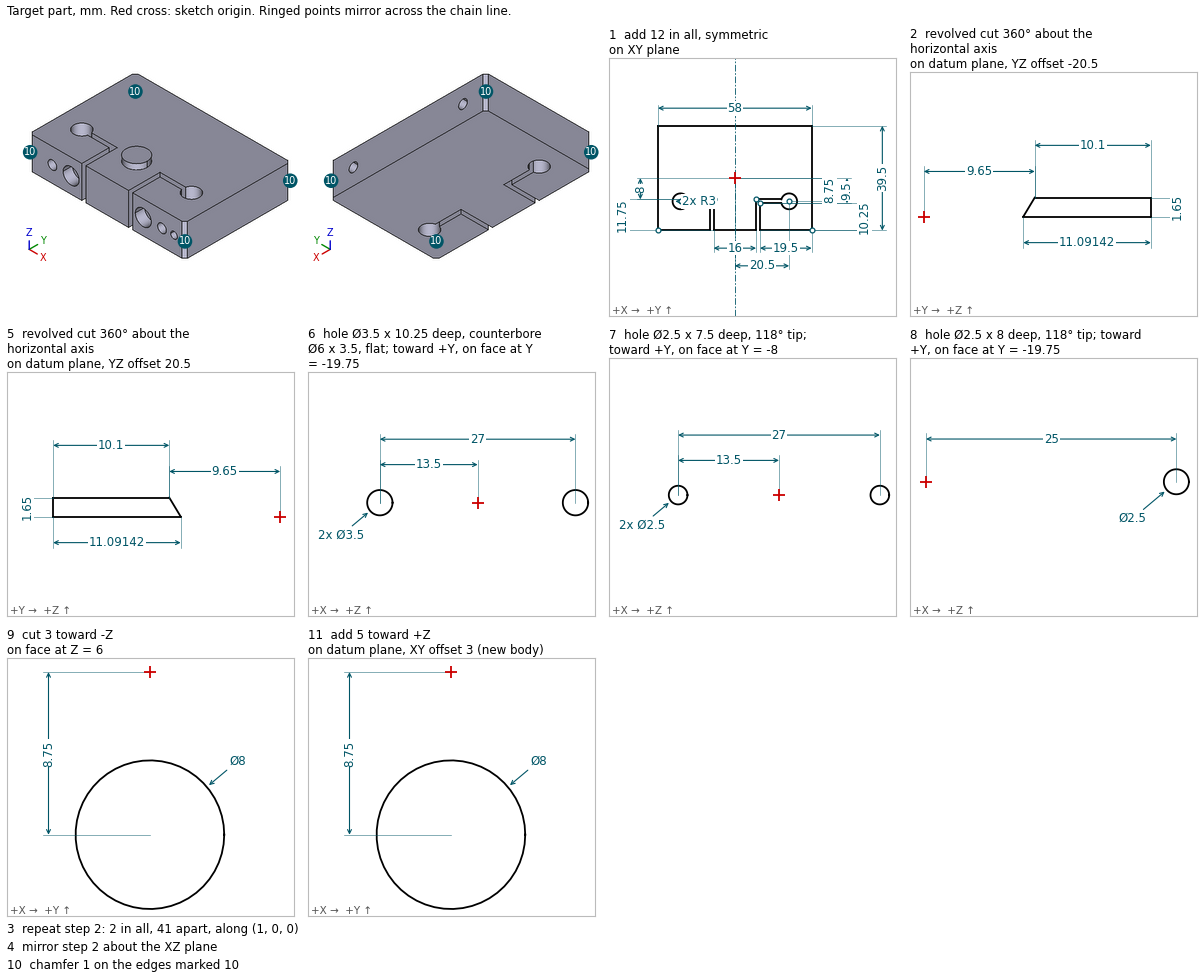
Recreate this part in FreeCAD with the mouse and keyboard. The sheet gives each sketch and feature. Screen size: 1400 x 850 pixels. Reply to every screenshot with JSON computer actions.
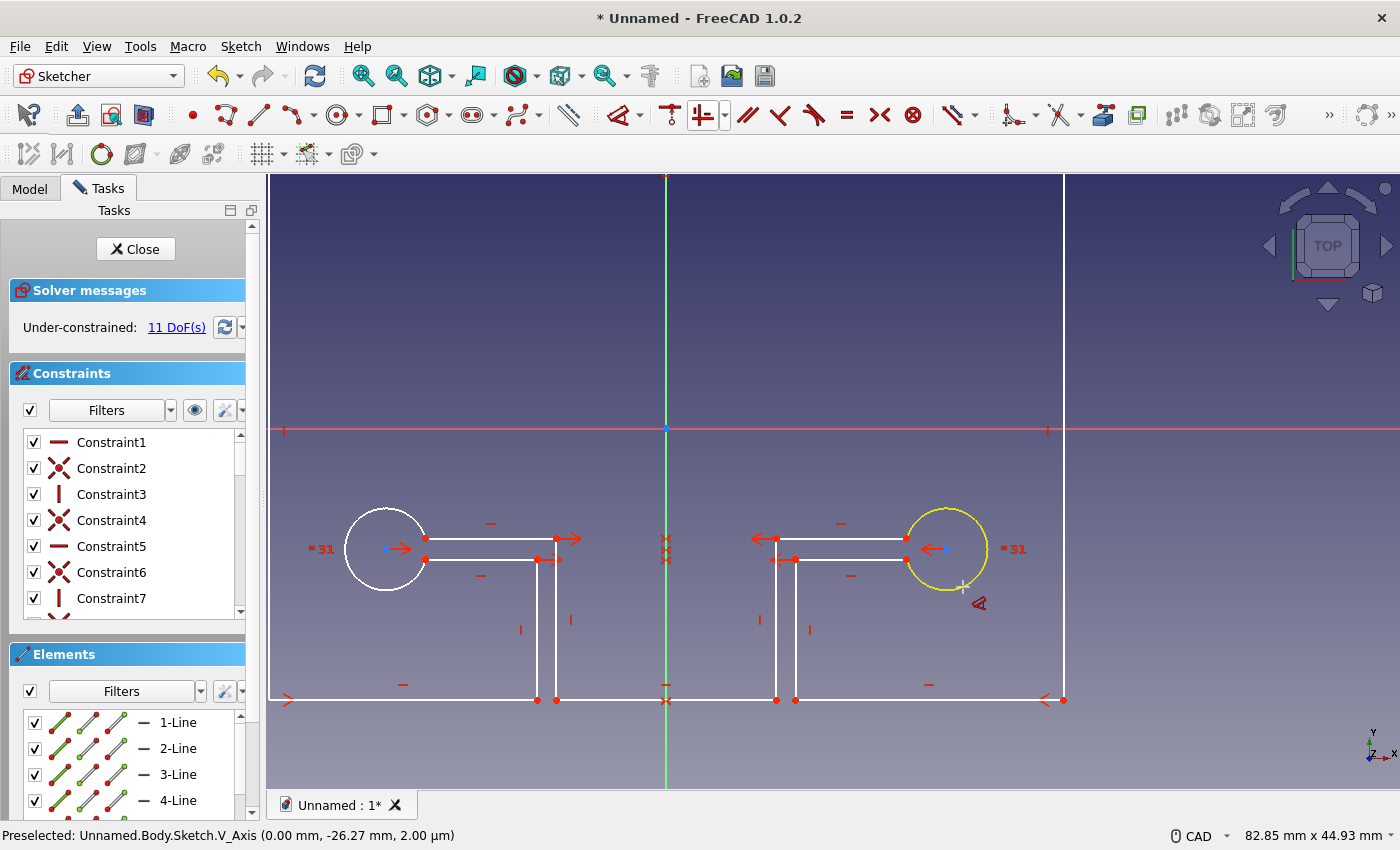
{"action": "left_click", "coordinate": [963, 587]}
{"action": "left_click", "coordinate": [976, 616]}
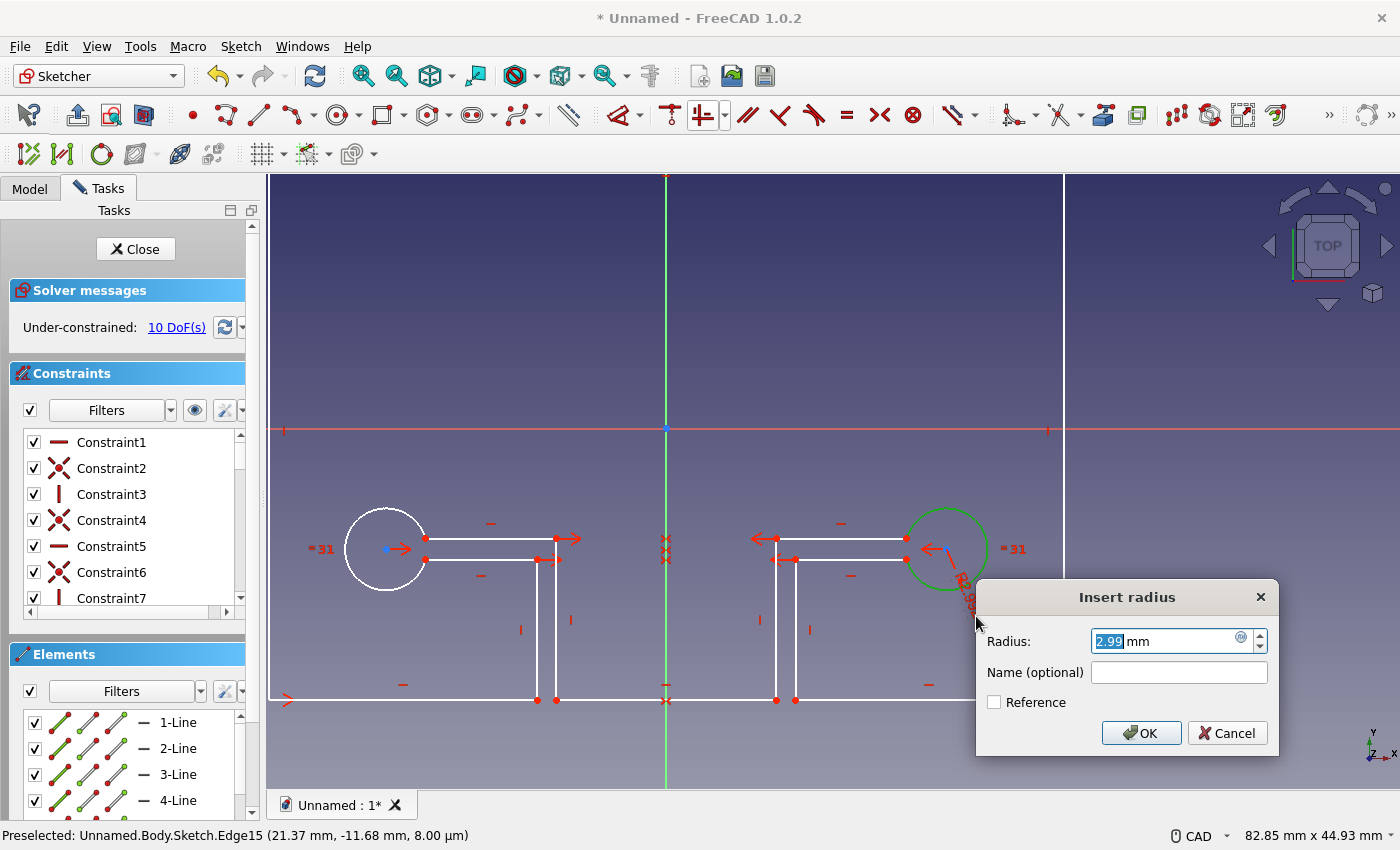
{"action": "type", "text": "3"}
{"action": "key", "text": "Return"}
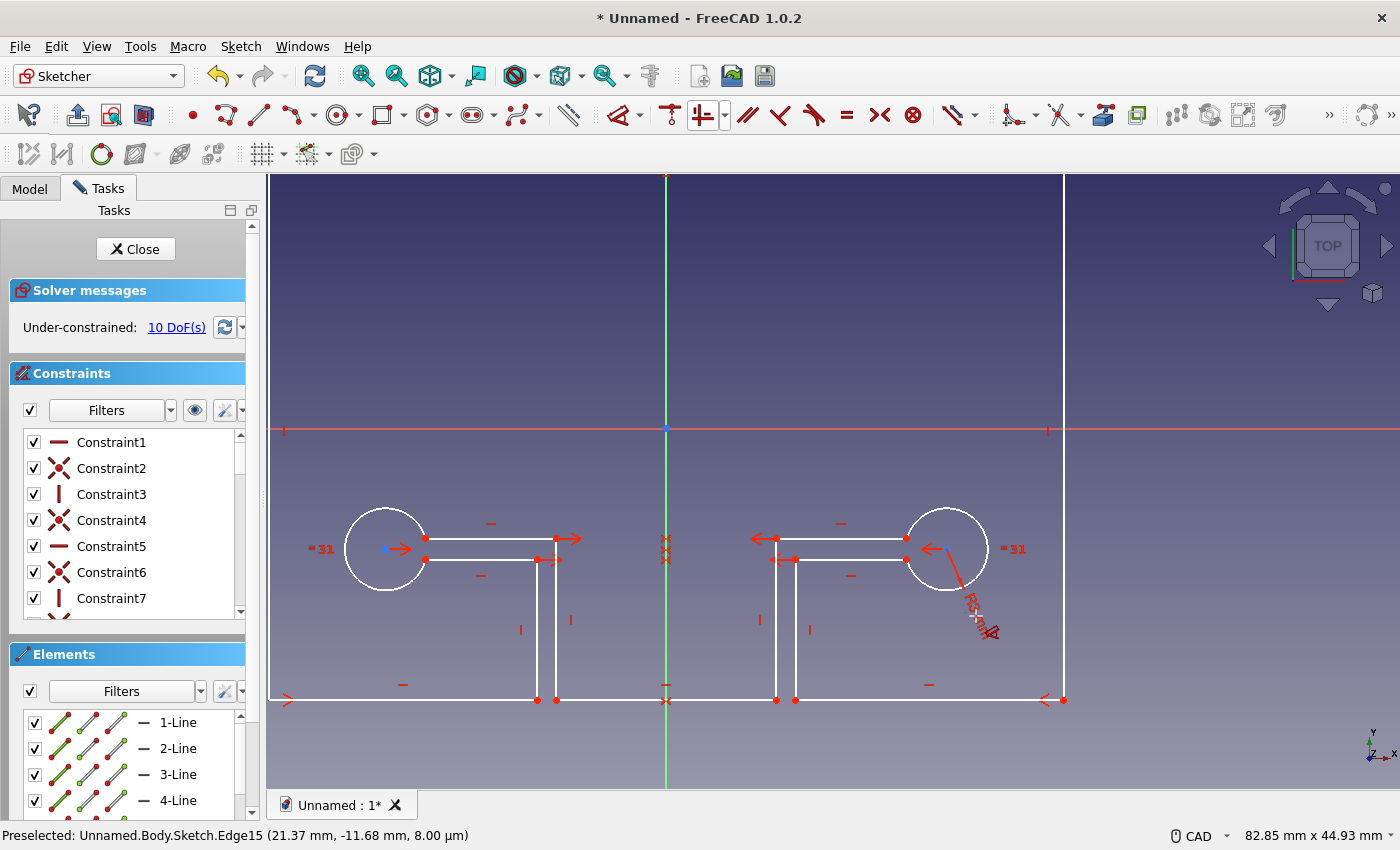
{"action": "left_click", "coordinate": [622, 700]}
{"action": "left_click", "coordinate": [616, 734]}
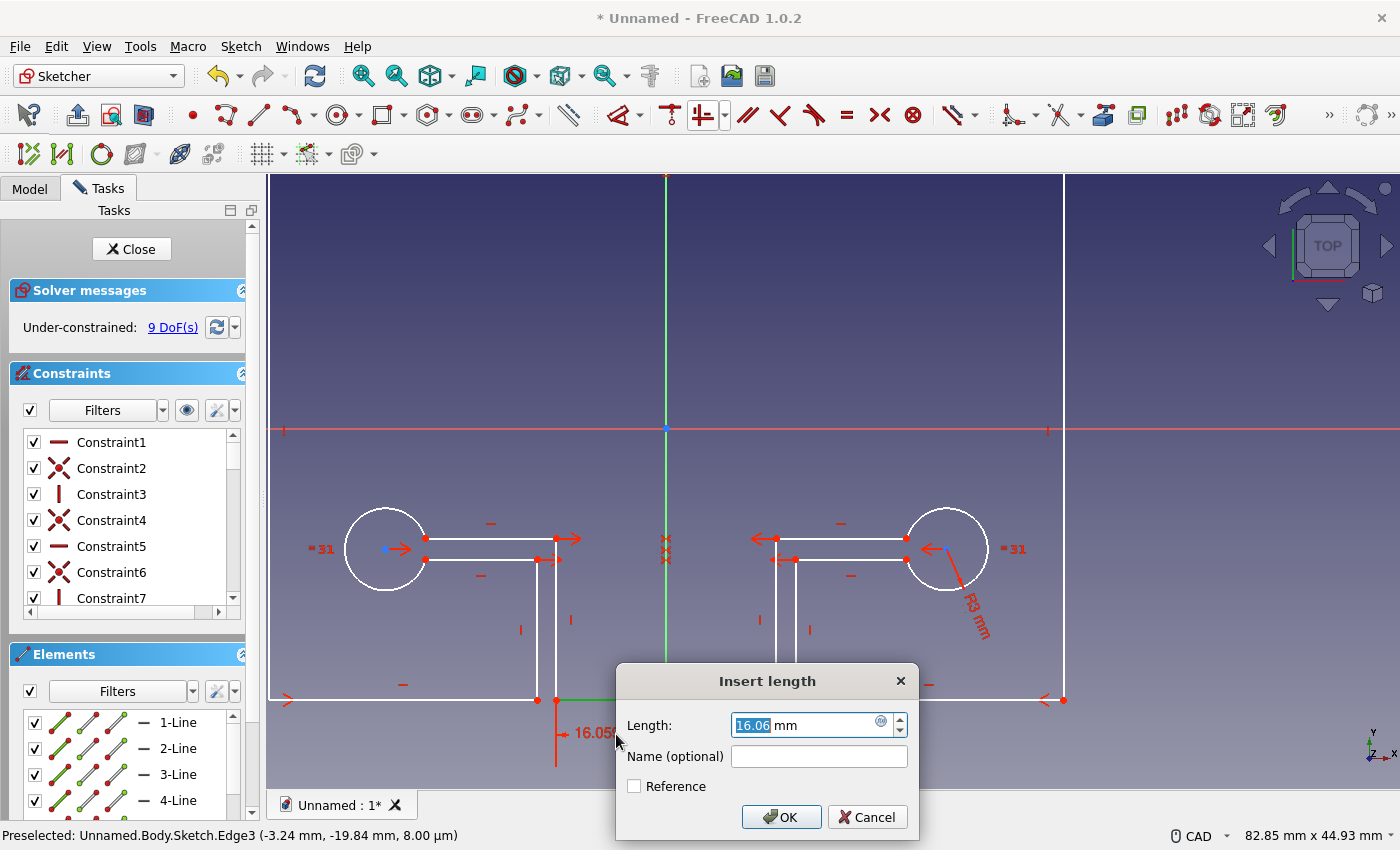
{"action": "type", "text": "16"}
{"action": "key", "text": "Return"}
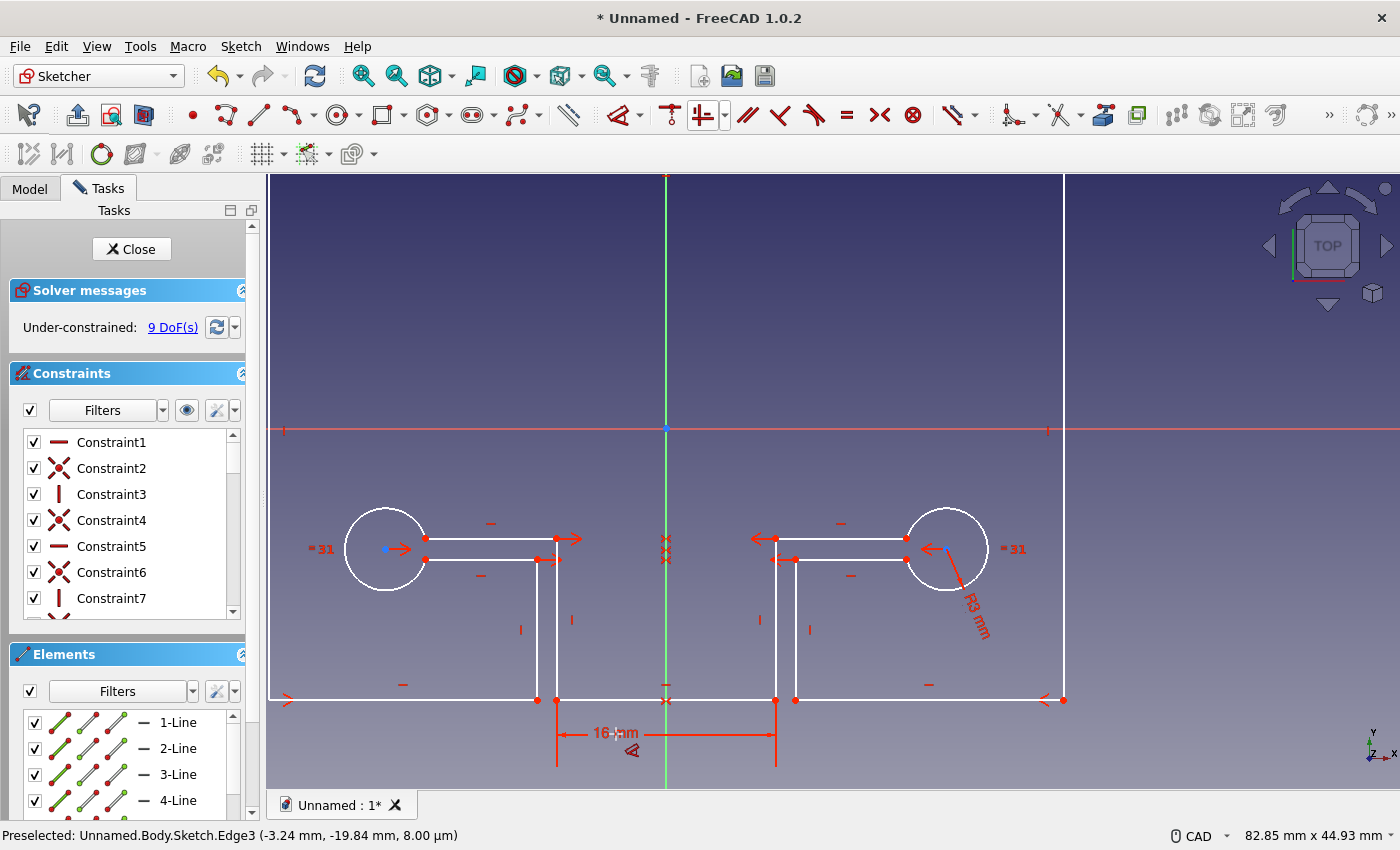
{"action": "scroll", "coordinate": [964, 589], "scroll_direction": "down", "scroll_amount": 2}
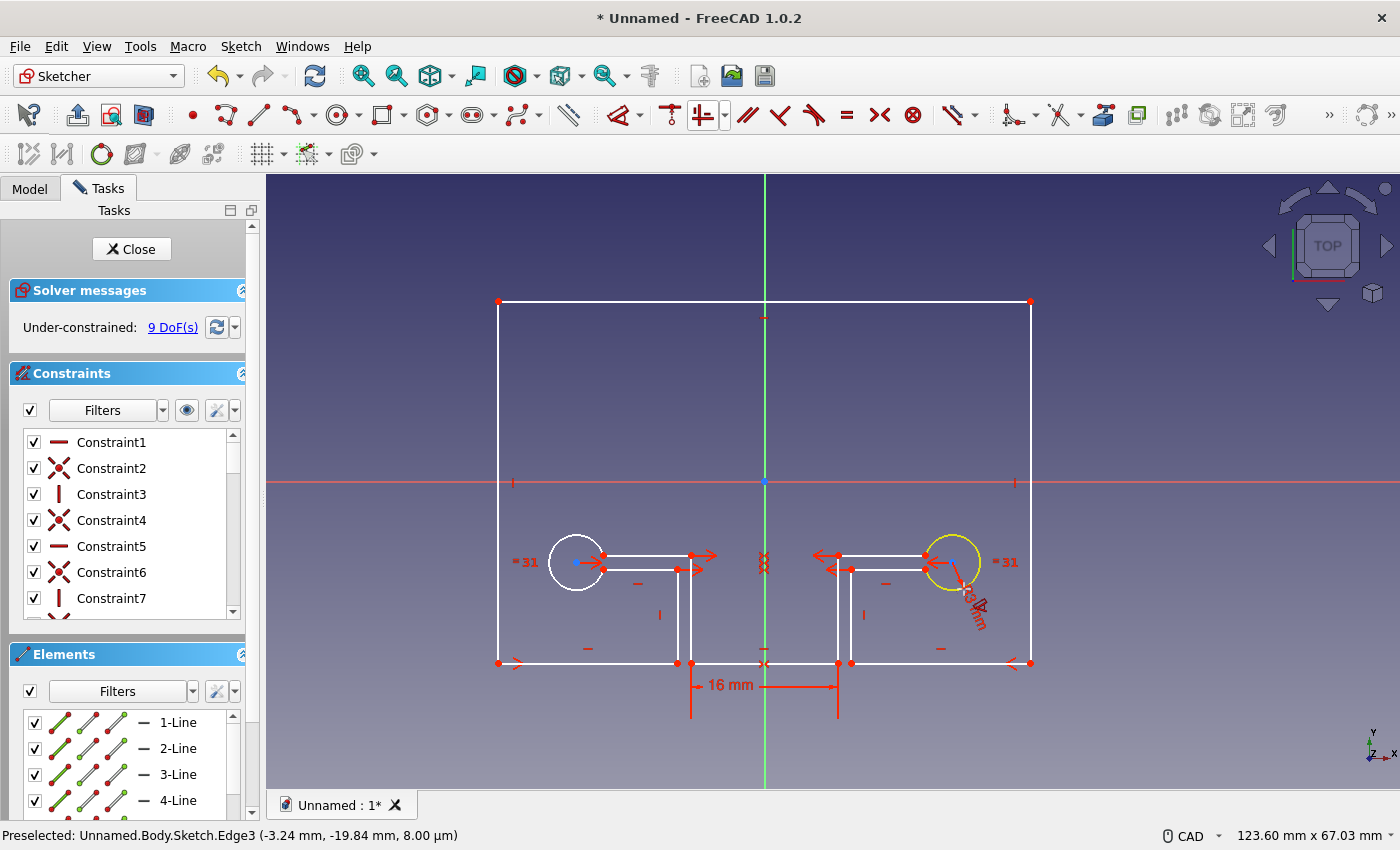
{"action": "left_click", "coordinate": [871, 302]}
{"action": "left_click", "coordinate": [642, 268]}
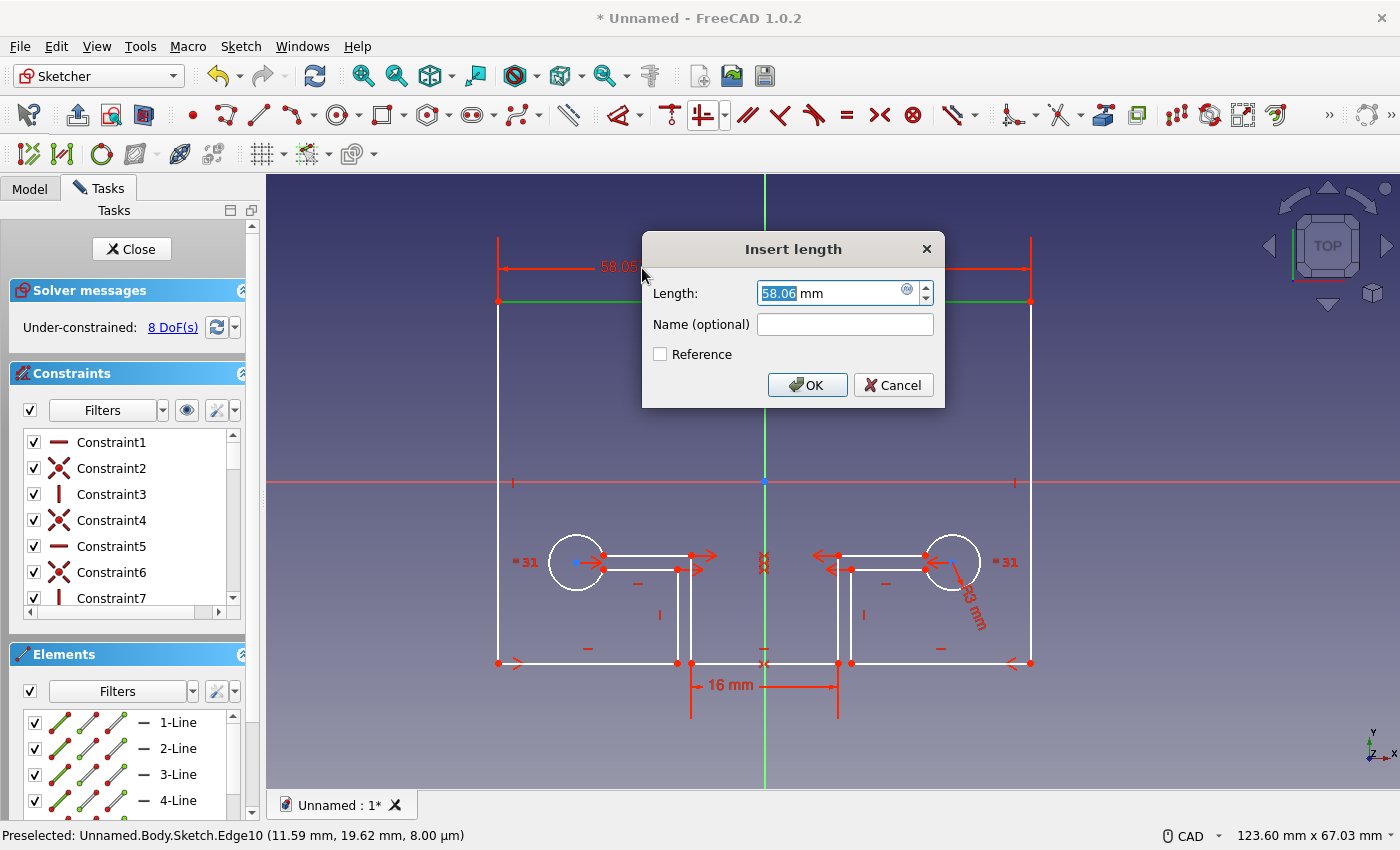
{"action": "type", "text": "58"}
{"action": "key", "text": "Return"}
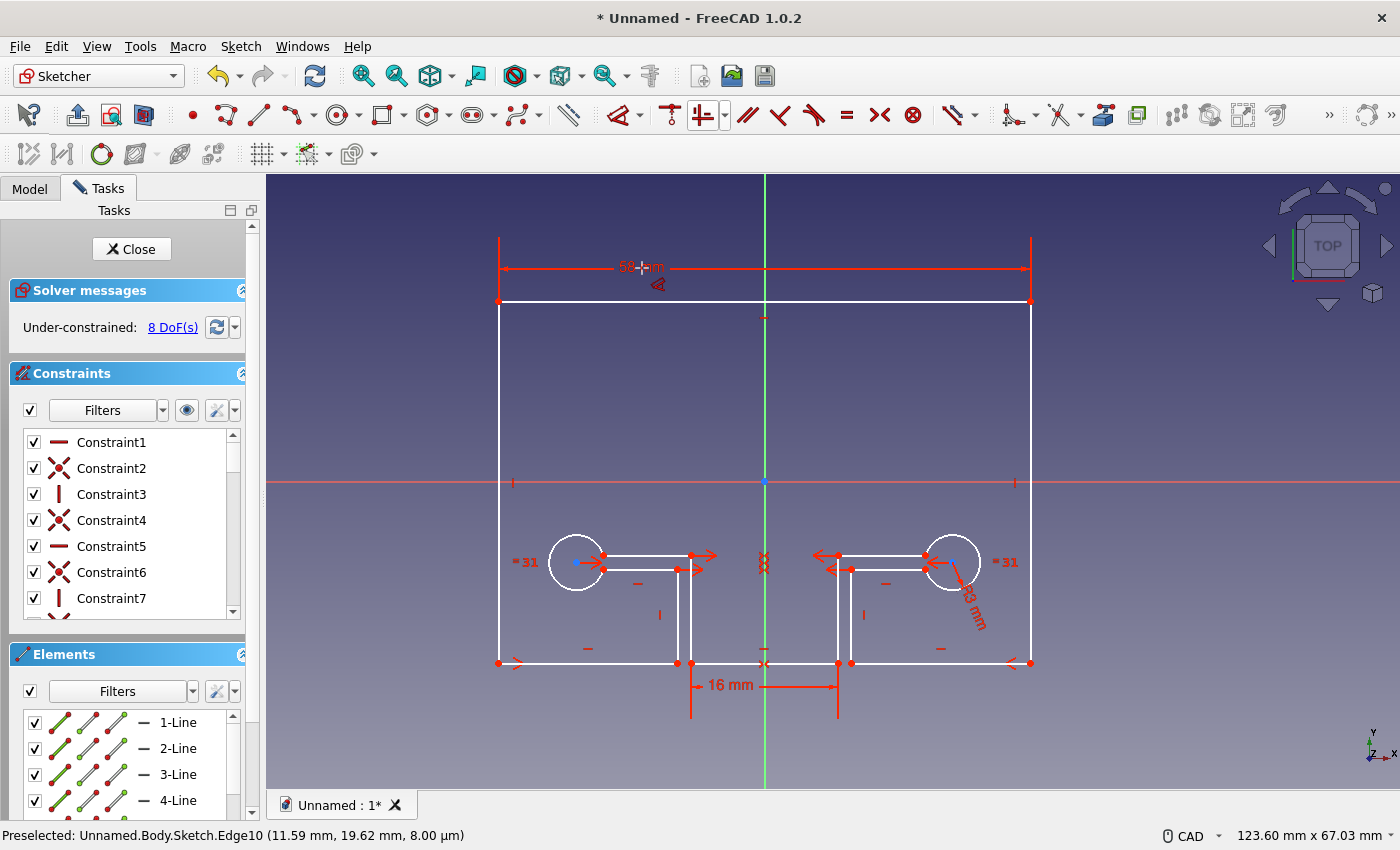
{"action": "left_click", "coordinate": [603, 556]}
{"action": "left_click", "coordinate": [569, 519]}